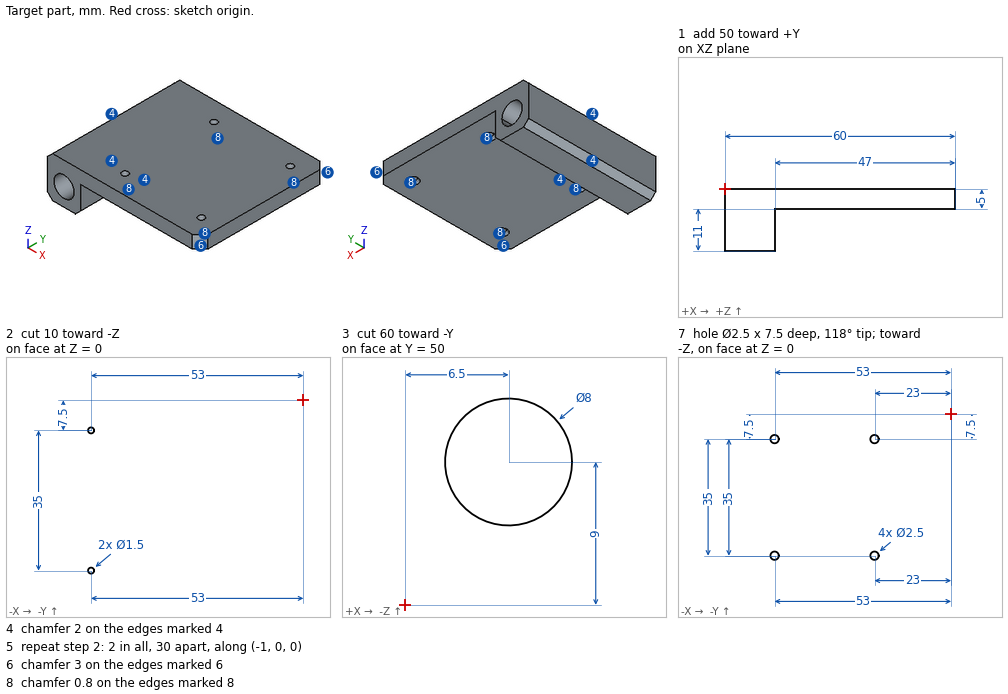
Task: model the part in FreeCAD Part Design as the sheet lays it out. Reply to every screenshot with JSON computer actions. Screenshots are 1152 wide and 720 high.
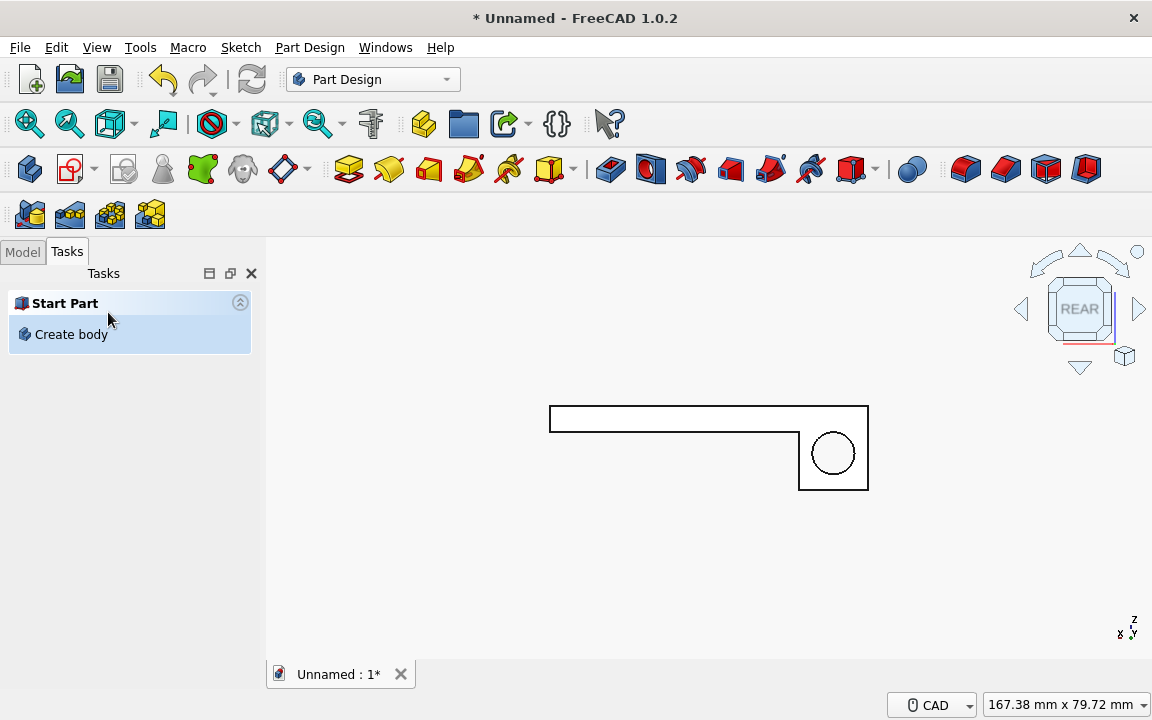
{"action": "key", "text": "0"}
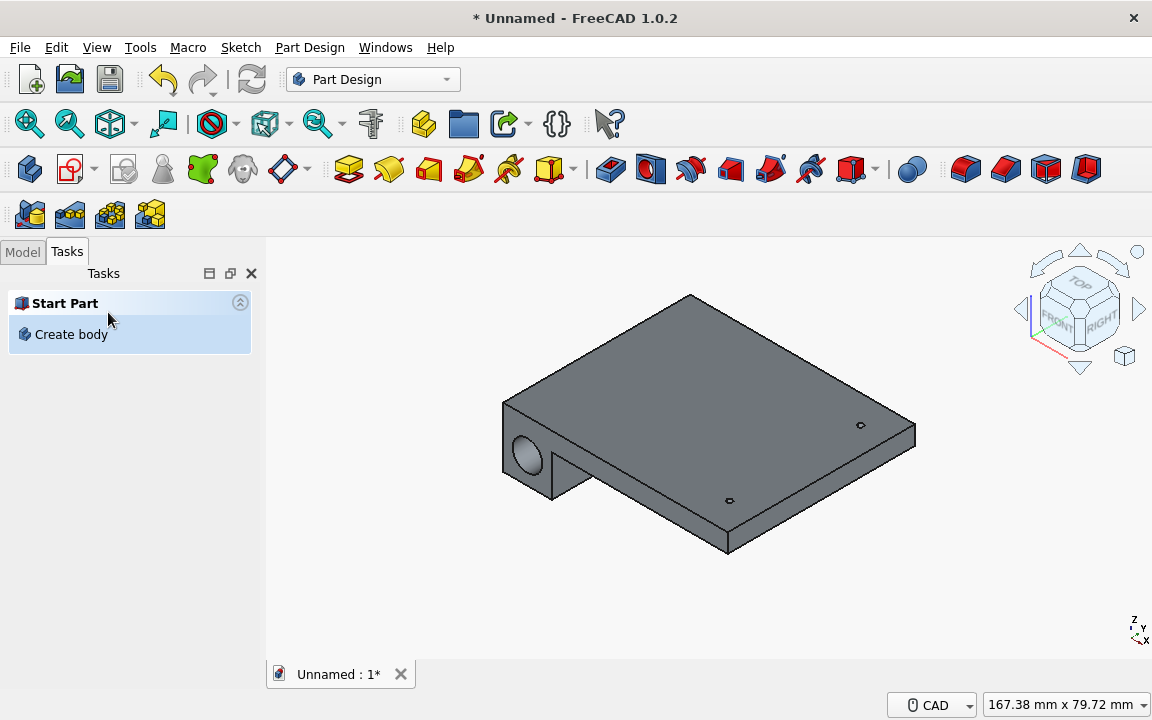
{"action": "key", "text": "2"}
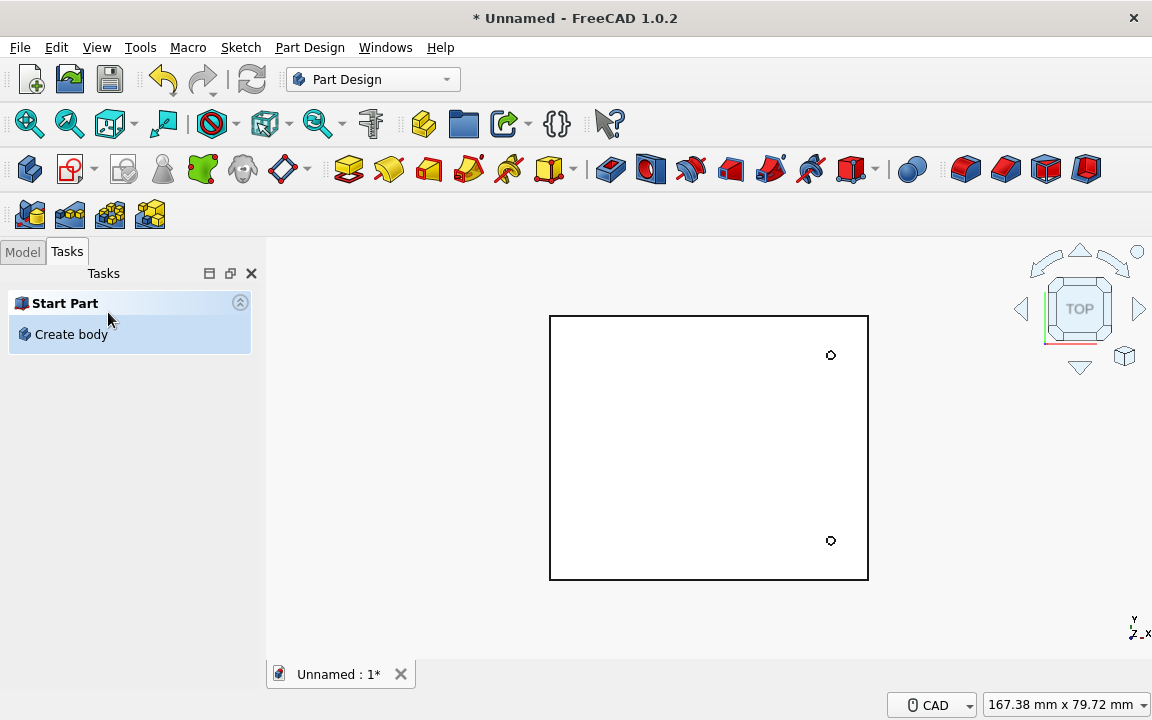
{"action": "key", "text": "1"}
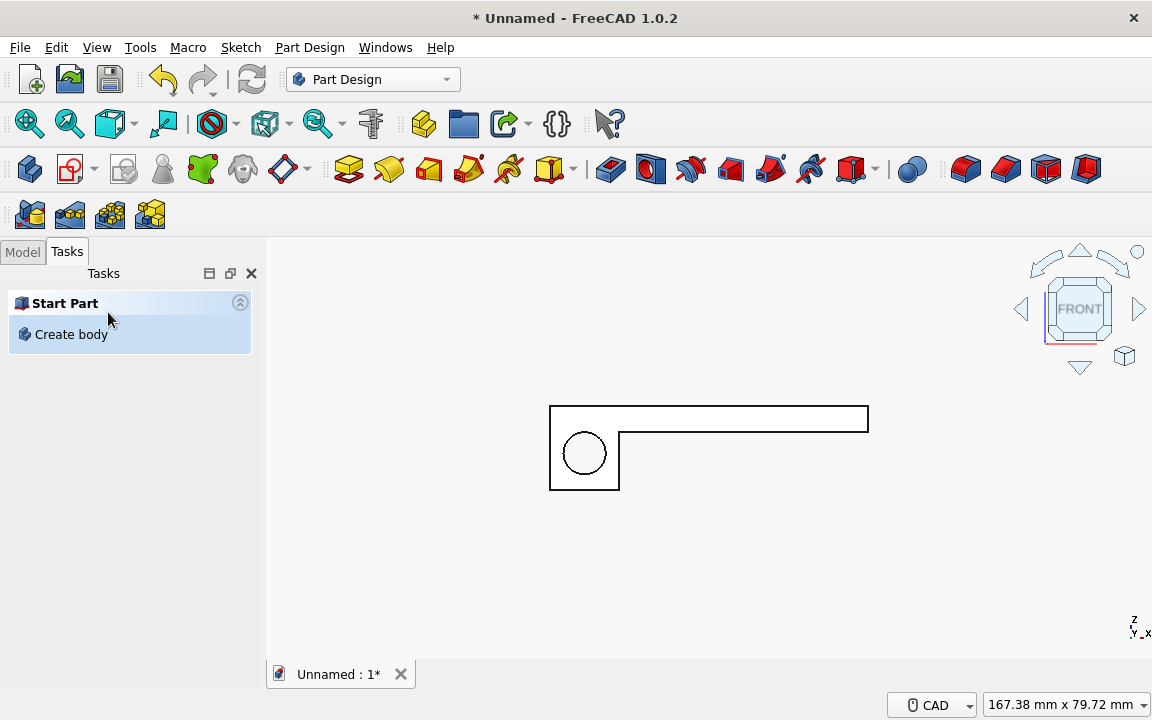
{"action": "left_click", "coordinate": [30, 124]}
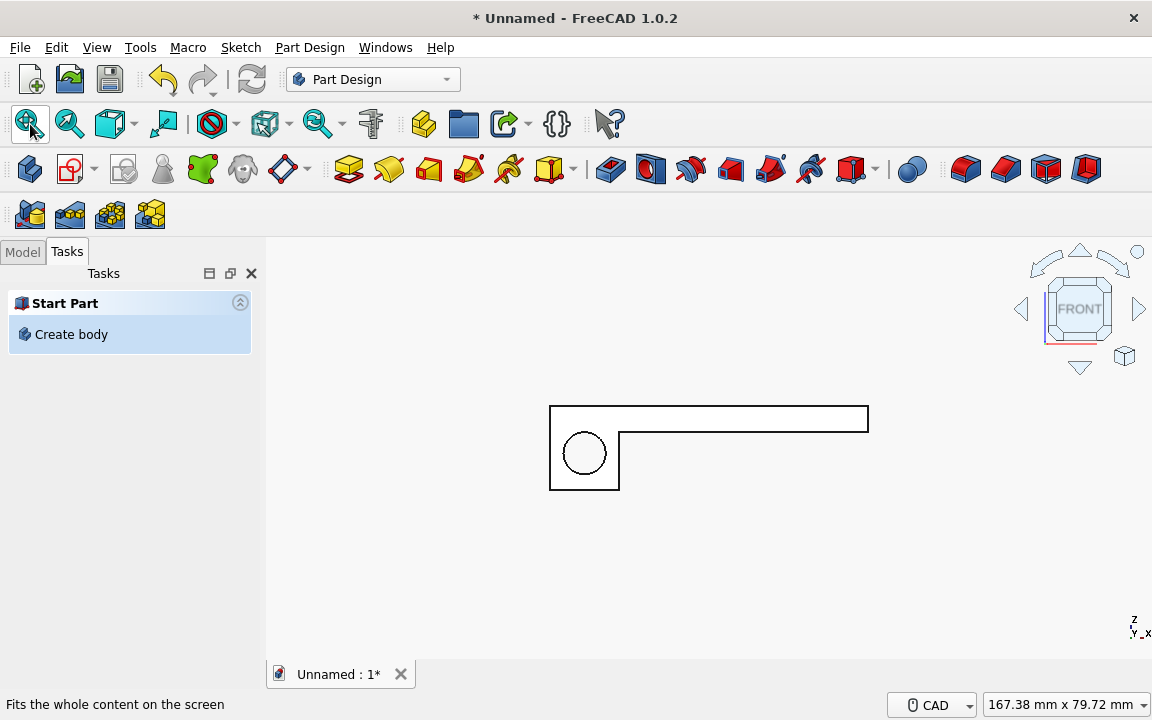
{"action": "key", "text": "3"}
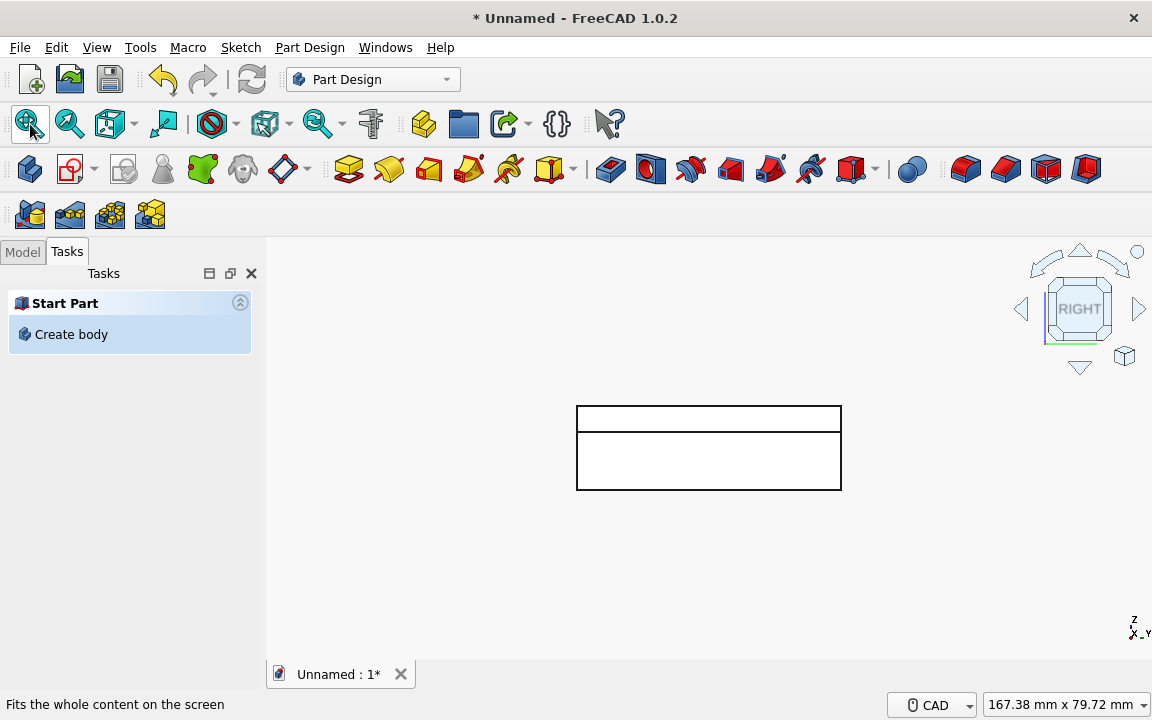
{"action": "left_click", "coordinate": [30, 124]}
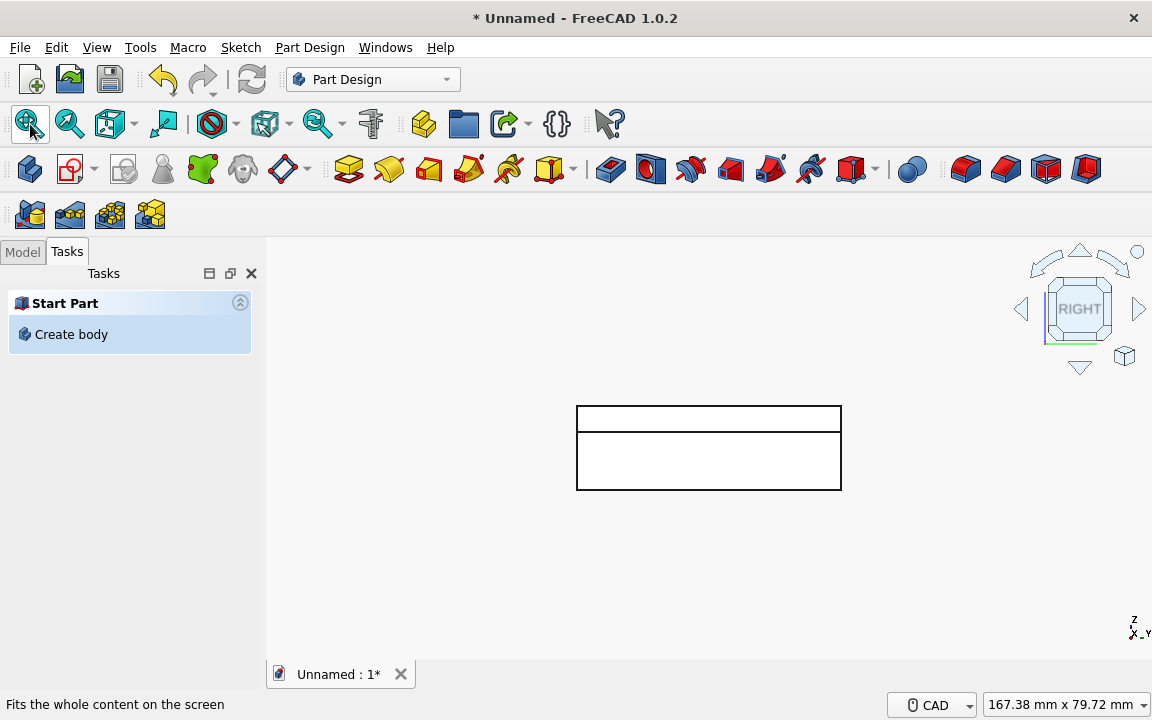
{"action": "left_click", "coordinate": [709, 489]}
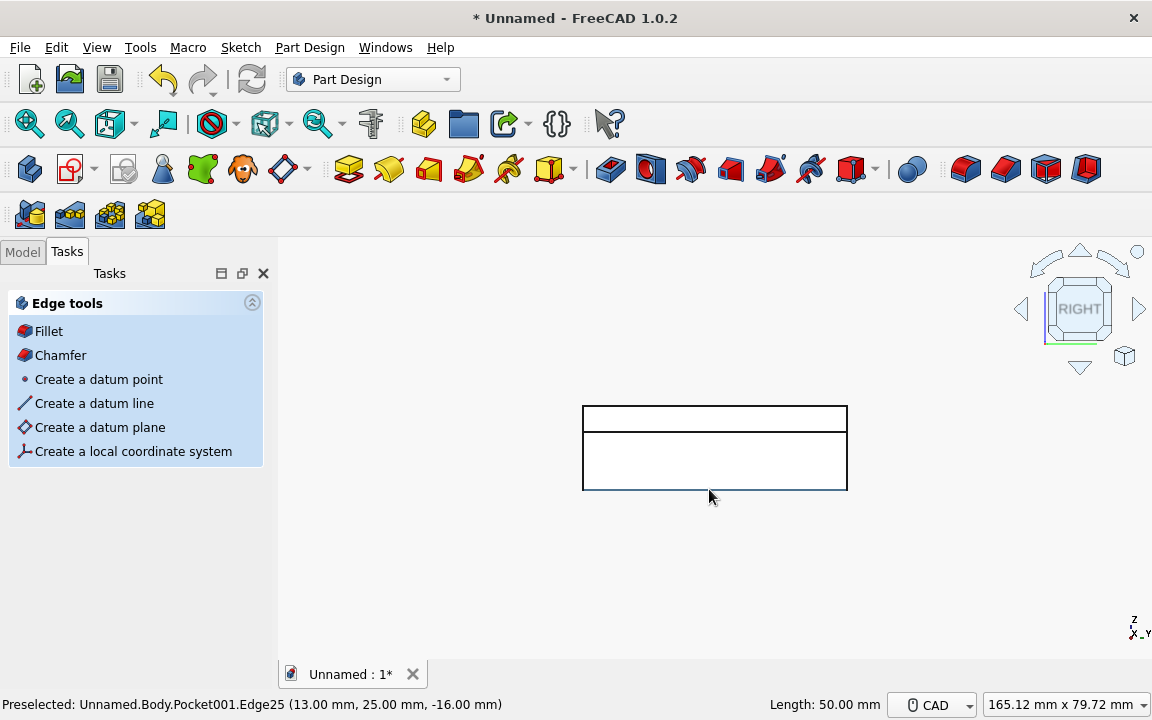
{"action": "key", "text": "5"}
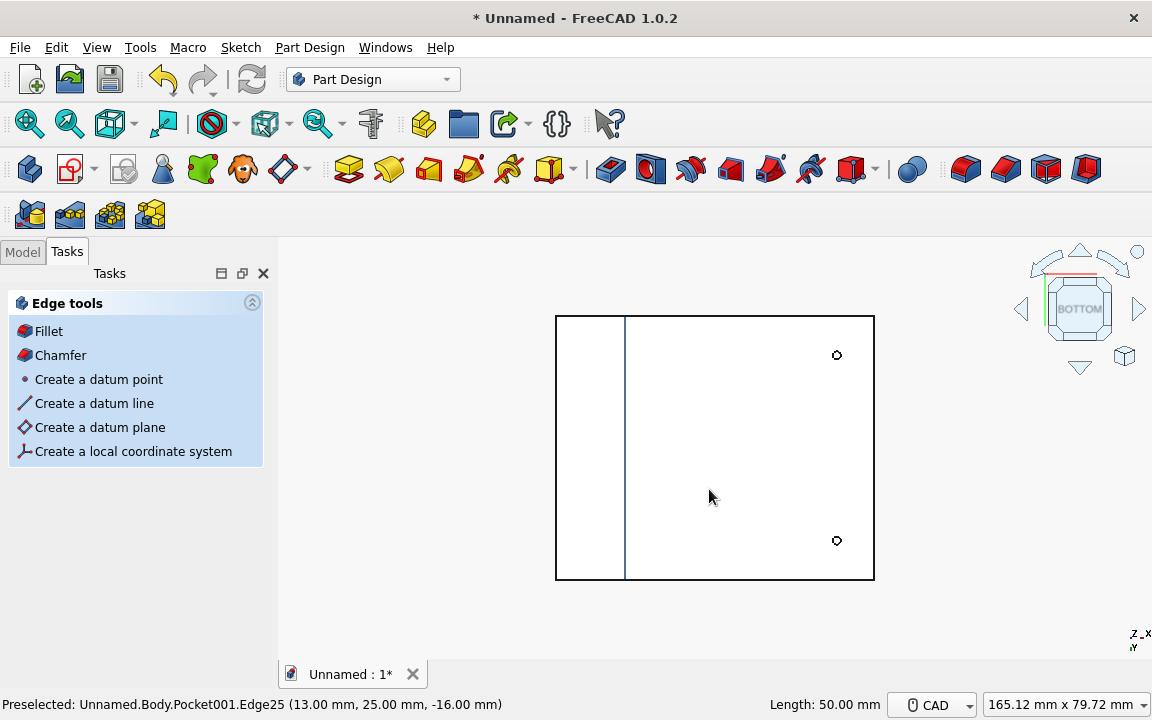
{"action": "left_click", "coordinate": [556, 447], "text": "ctrl"}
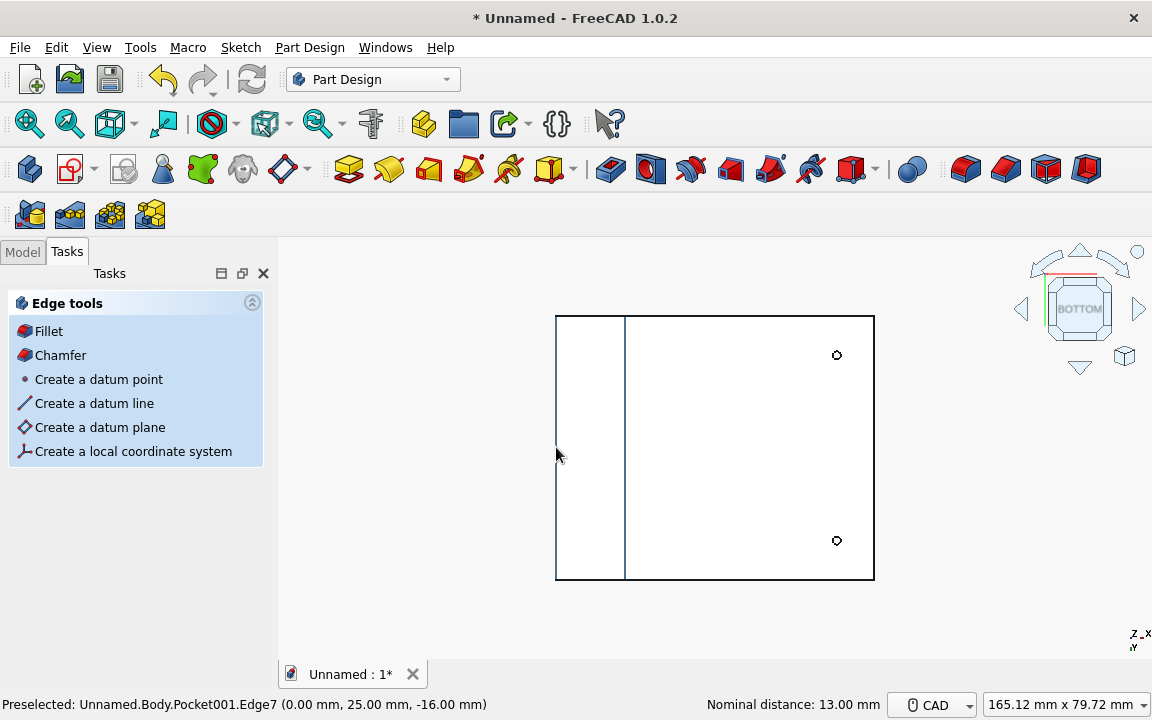
{"action": "key", "text": "4"}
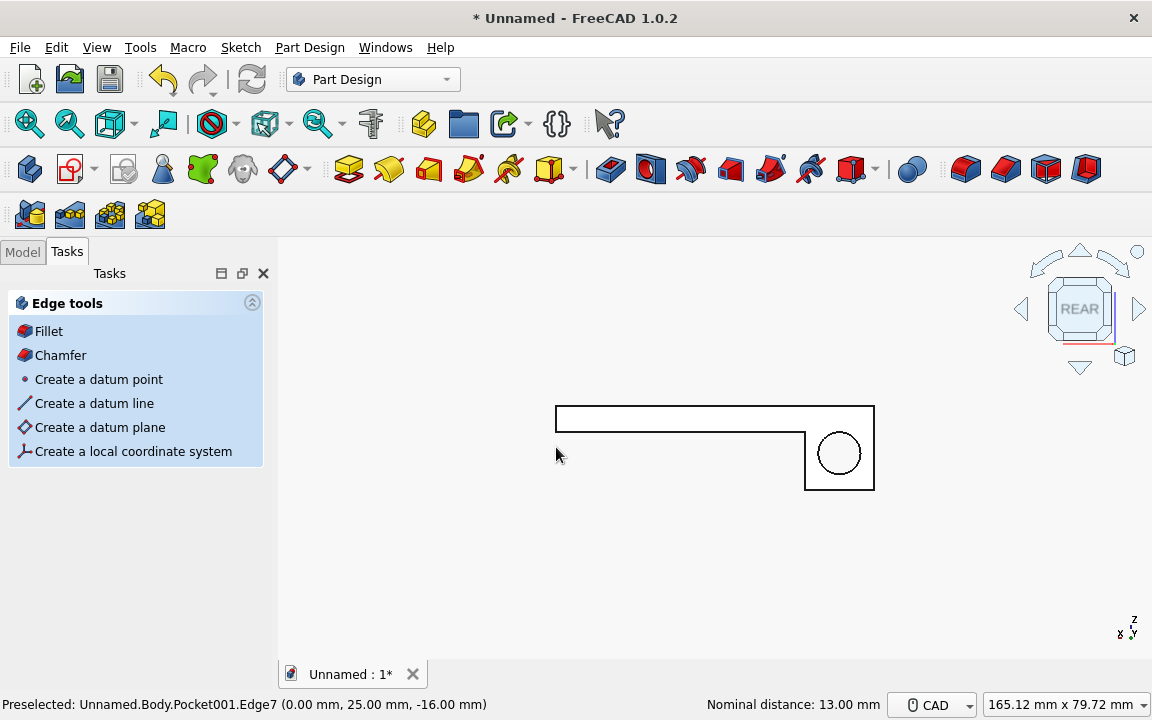
{"action": "key", "text": "v f"}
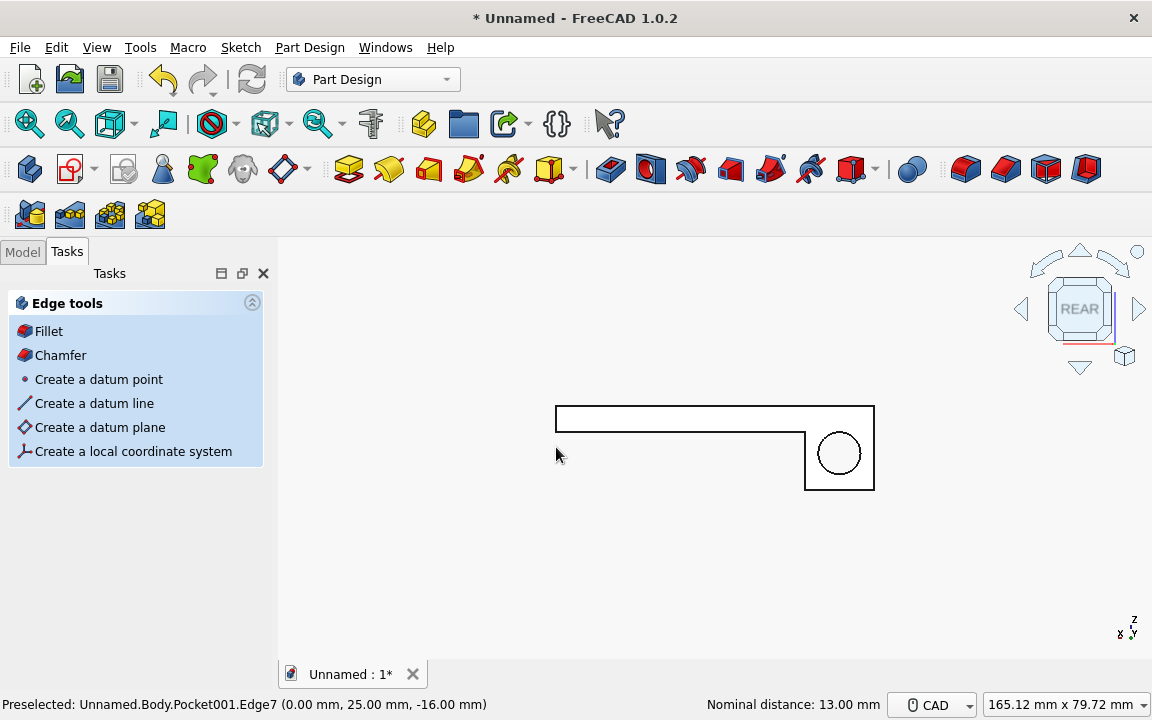
{"action": "key", "text": "6"}